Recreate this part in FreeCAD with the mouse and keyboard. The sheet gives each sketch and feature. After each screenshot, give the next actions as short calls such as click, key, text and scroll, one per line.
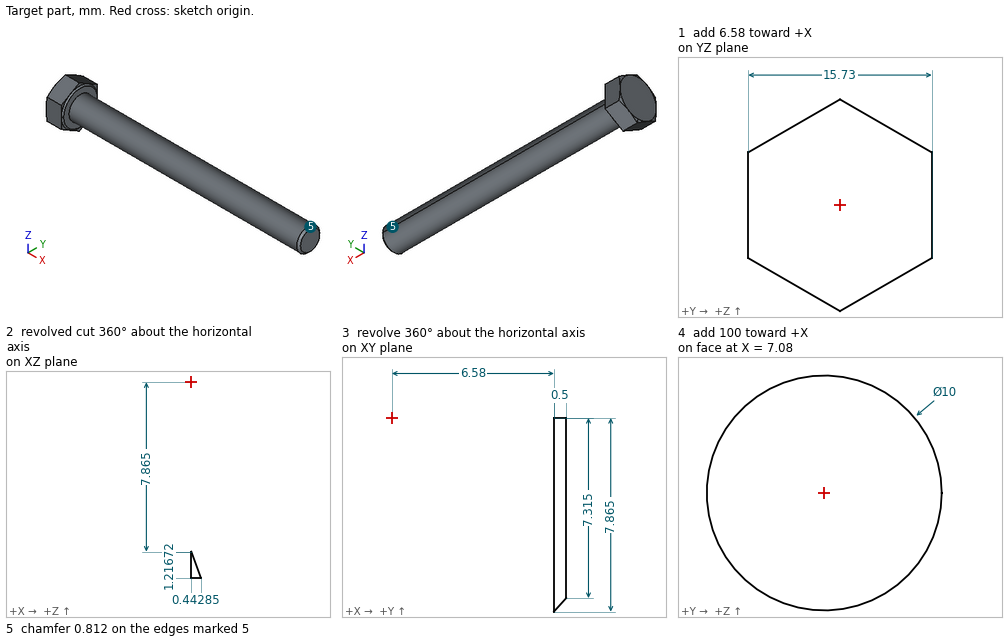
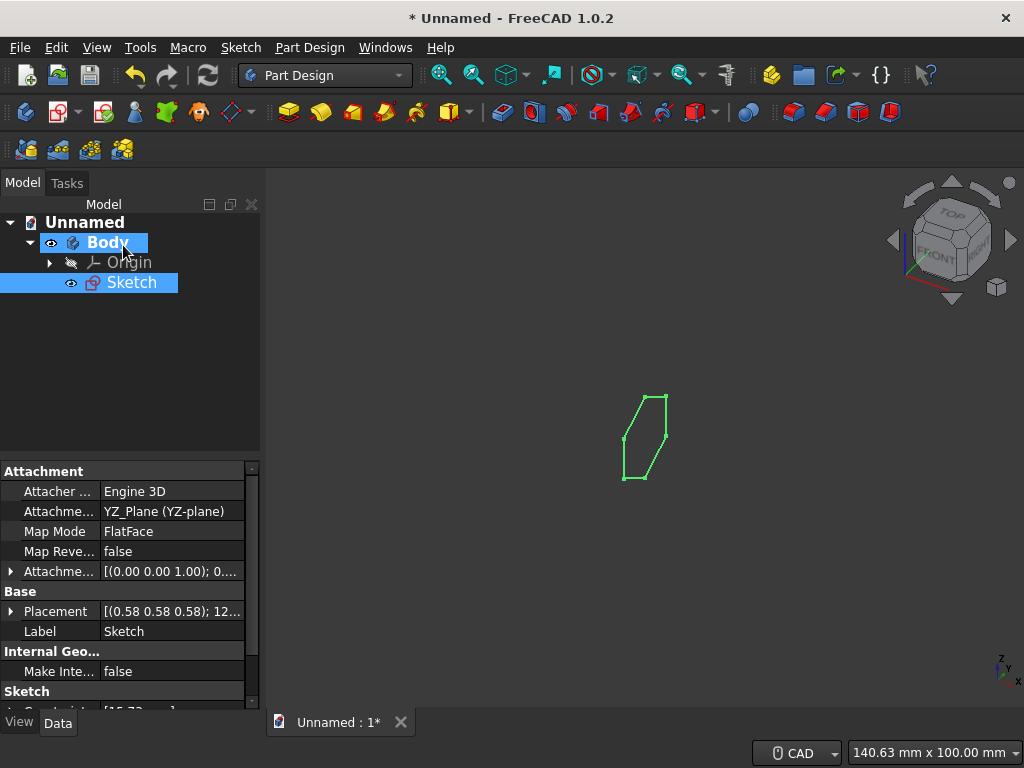
click(290, 112)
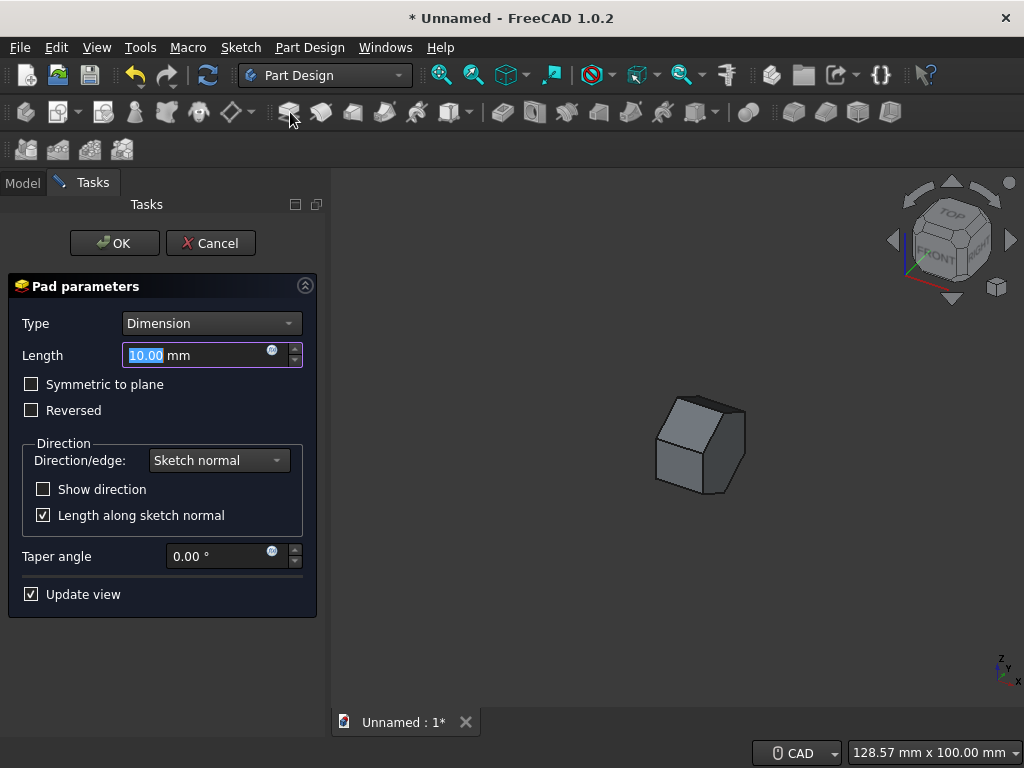
text(6.58)
key(Tab)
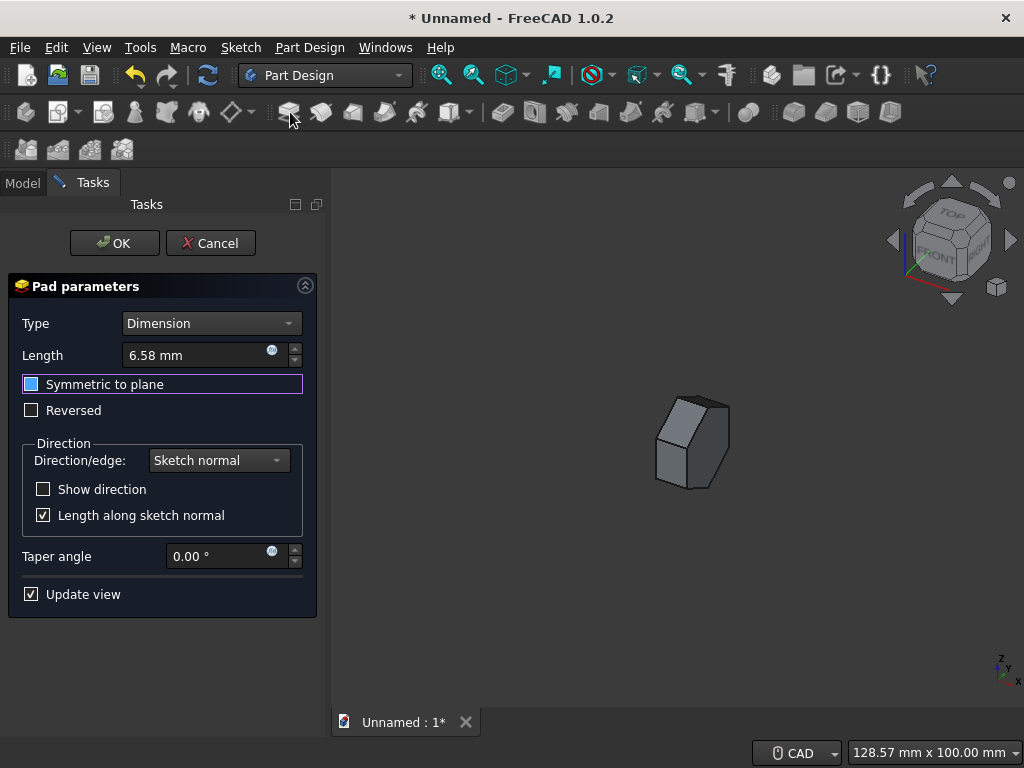
click(115, 243)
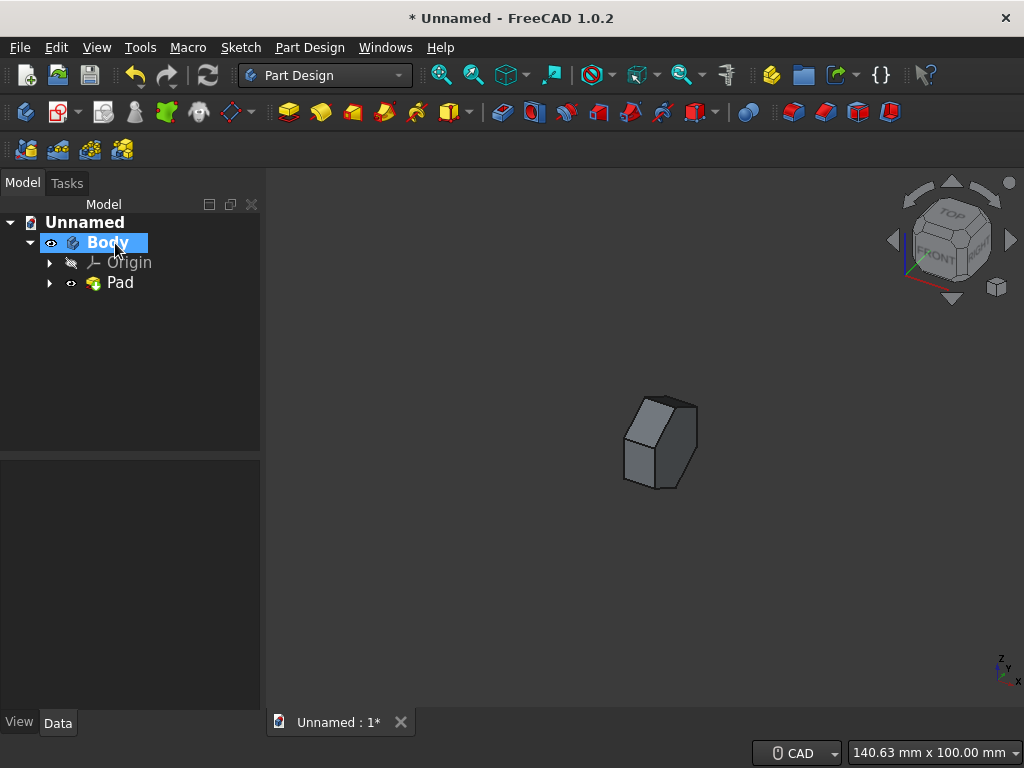
key(v)
key(f)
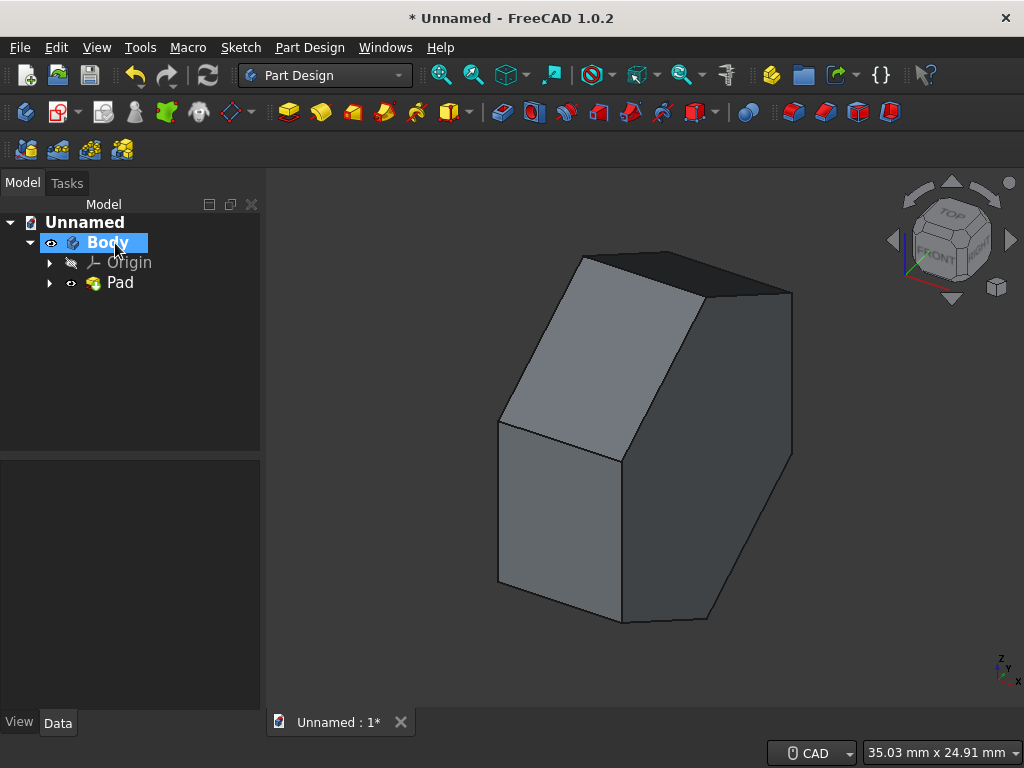
click(58, 112)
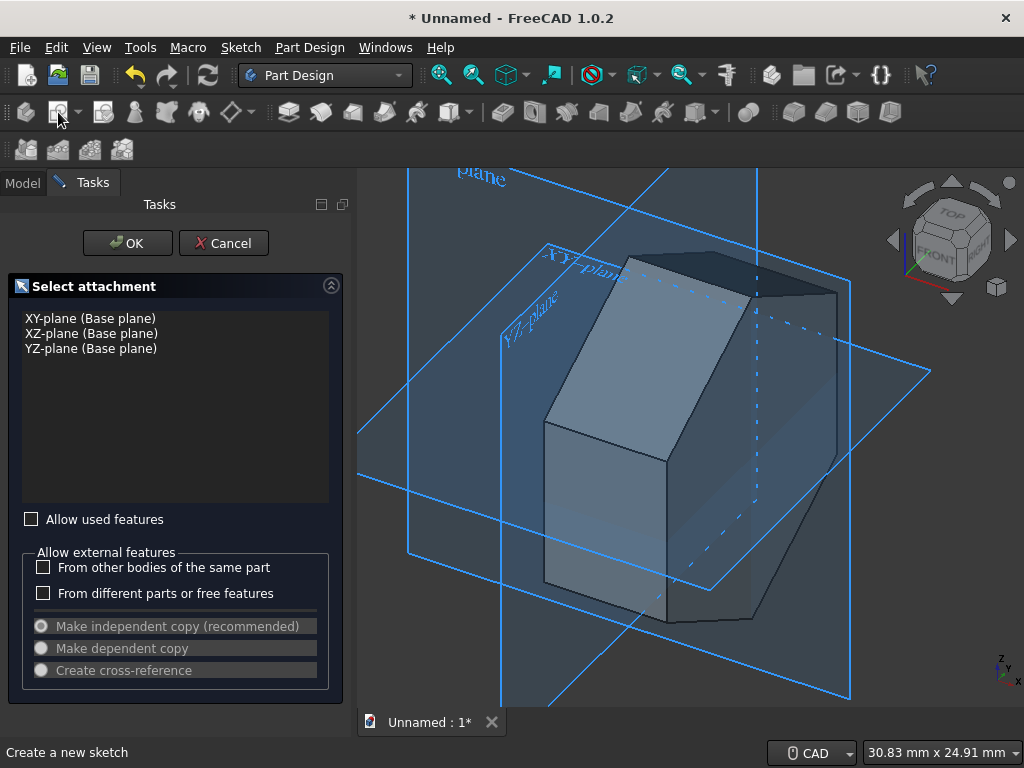
click(82, 334)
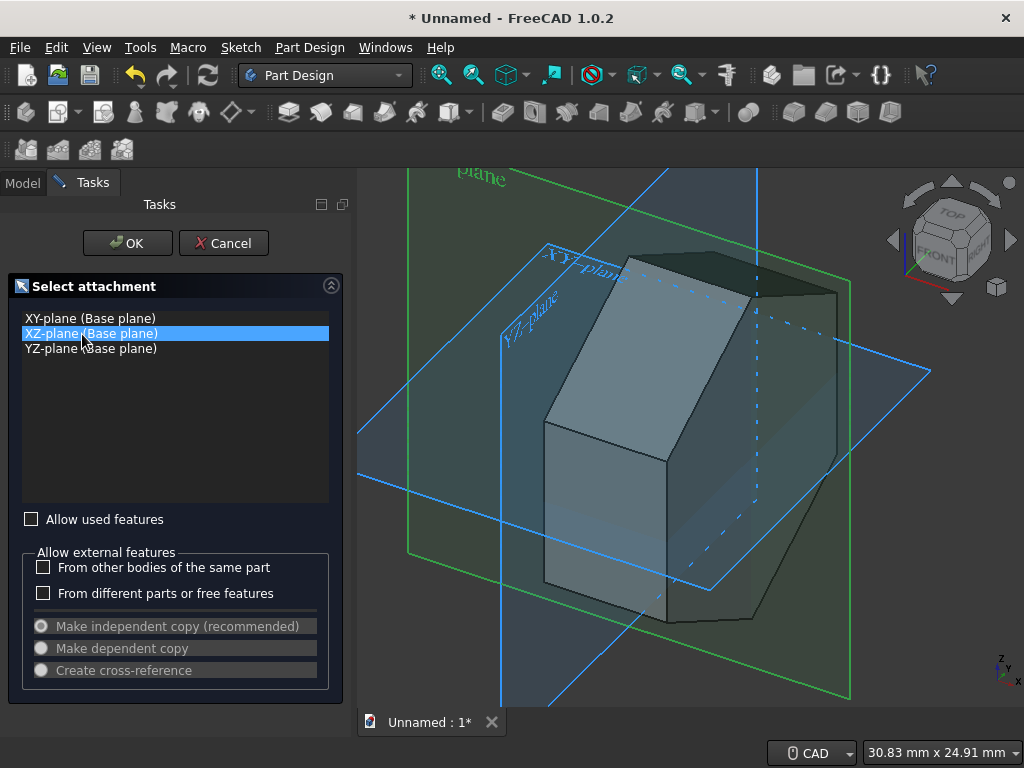
click(128, 243)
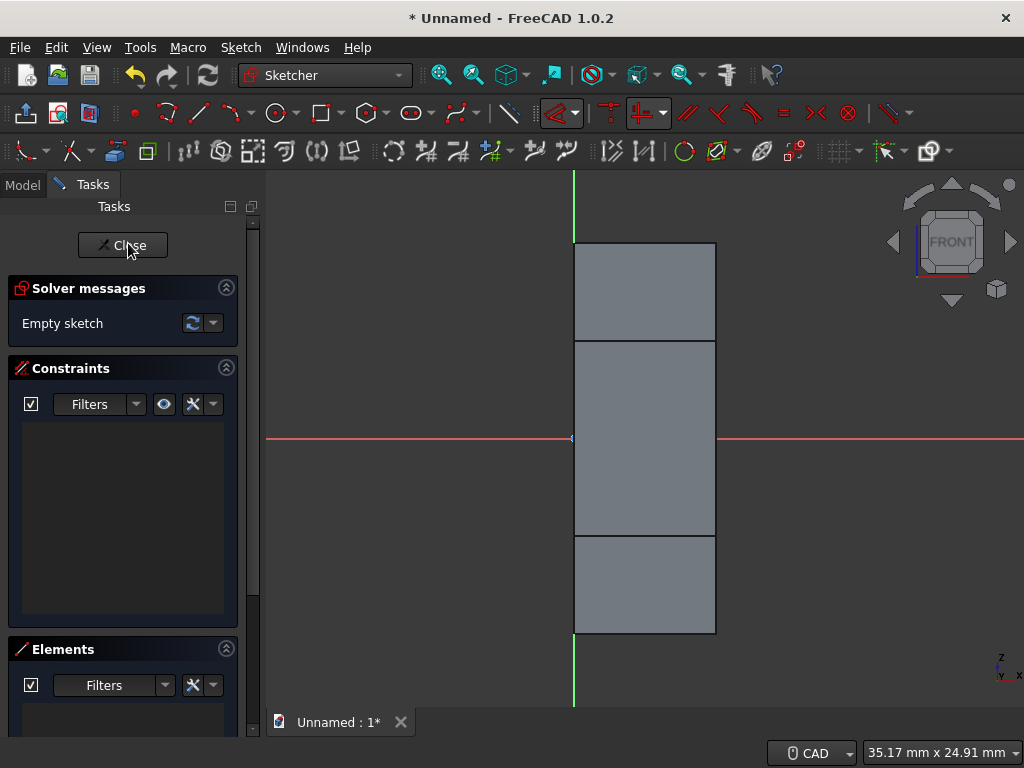
click(90, 114)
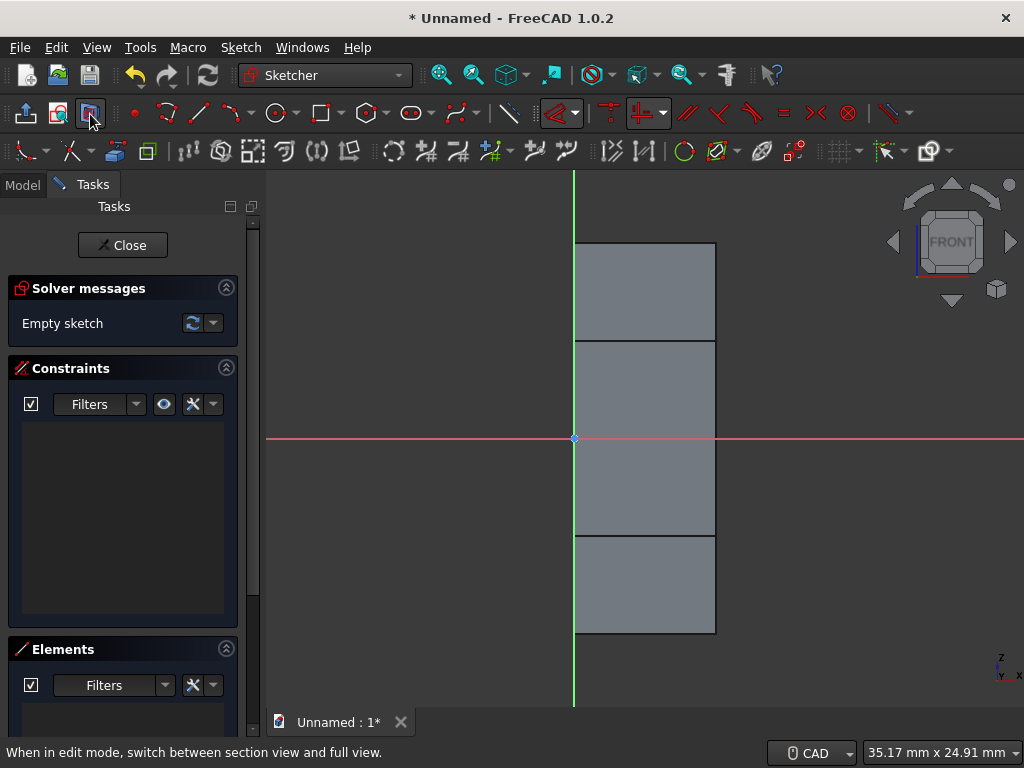
scroll(579, 636, up, 13)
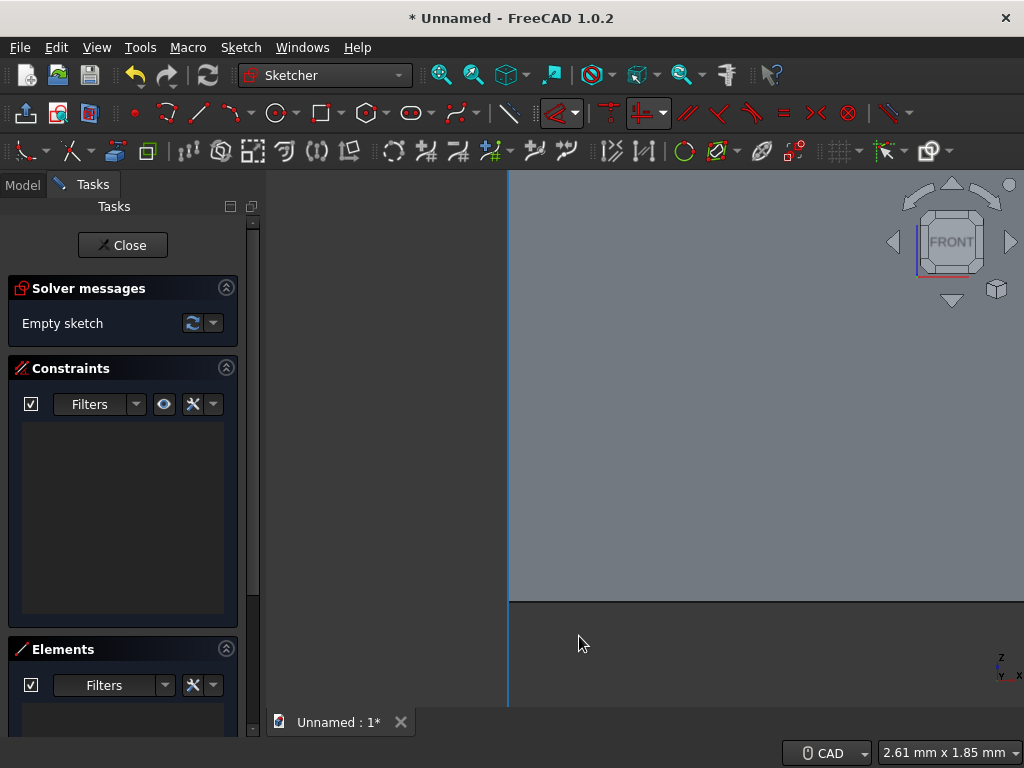
click(168, 114)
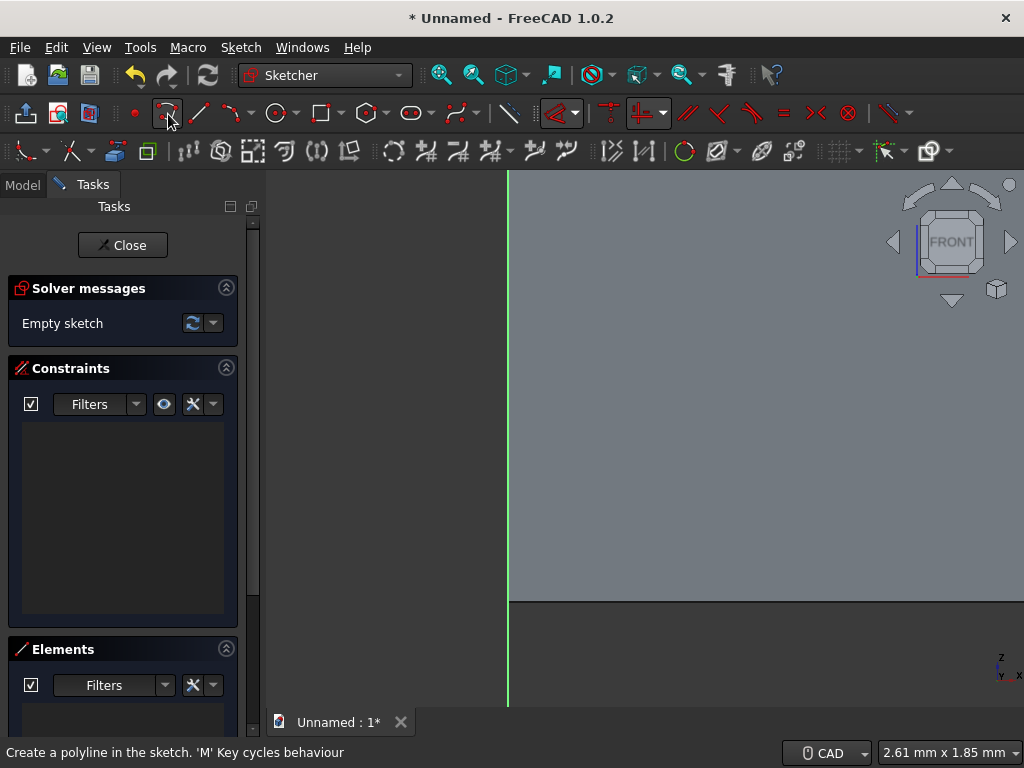
click(508, 249)
click(636, 602)
click(517, 602)
click(508, 250)
key(Escape)
key(Escape)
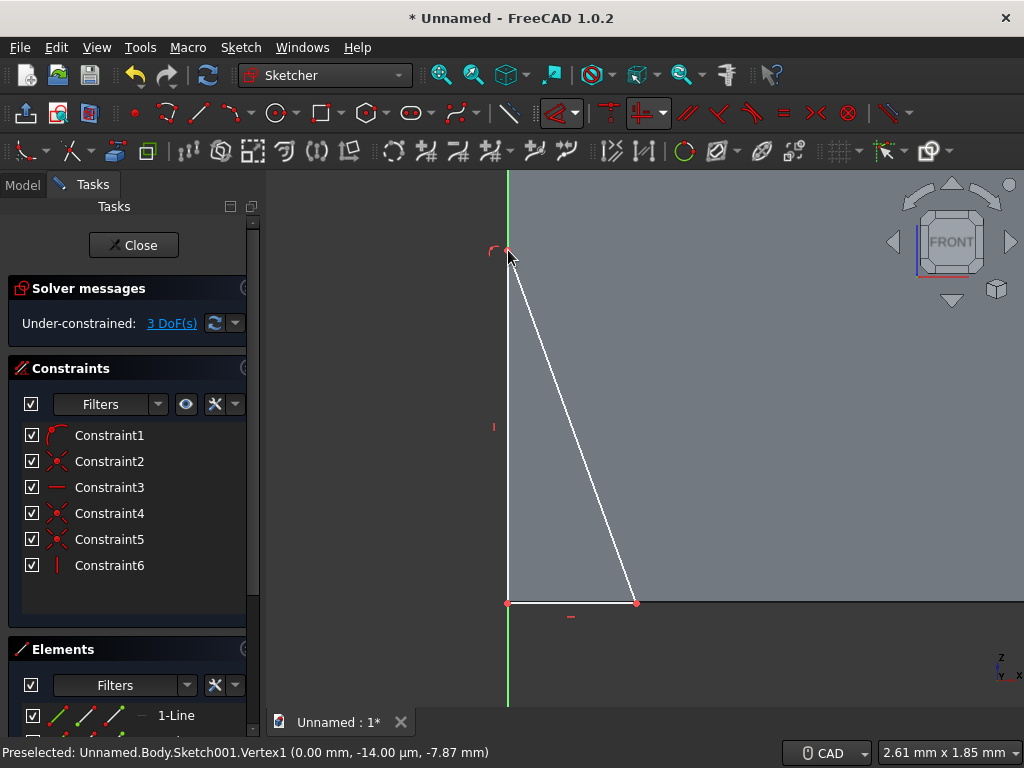
key(d)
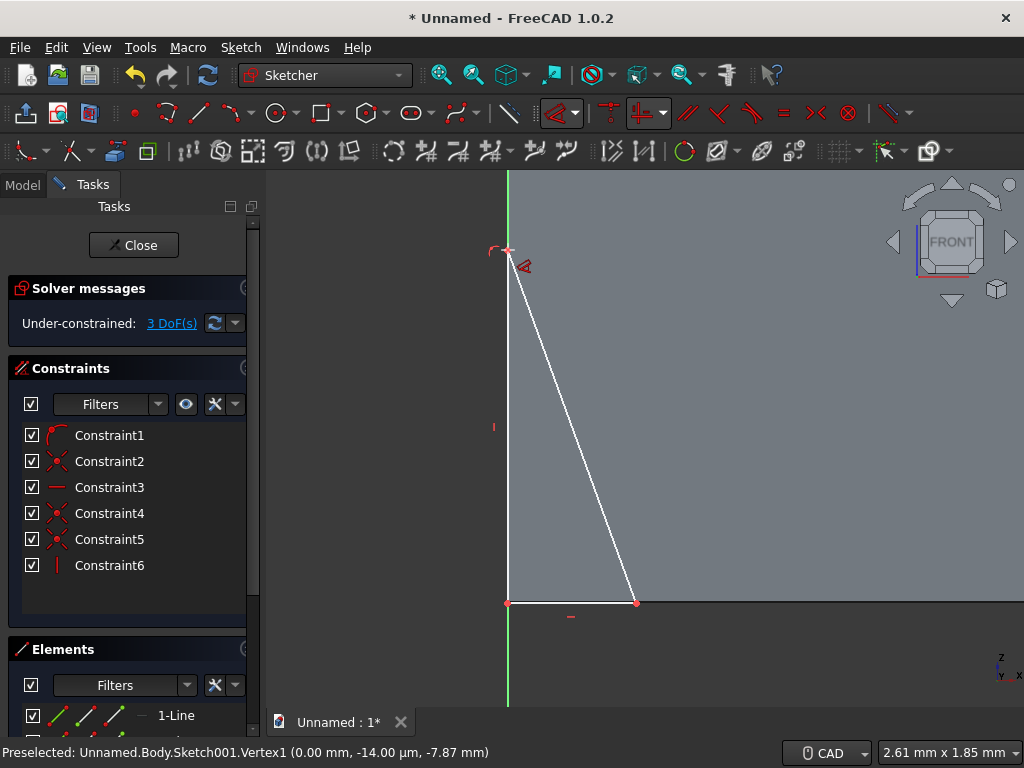
click(508, 250)
click(474, 224)